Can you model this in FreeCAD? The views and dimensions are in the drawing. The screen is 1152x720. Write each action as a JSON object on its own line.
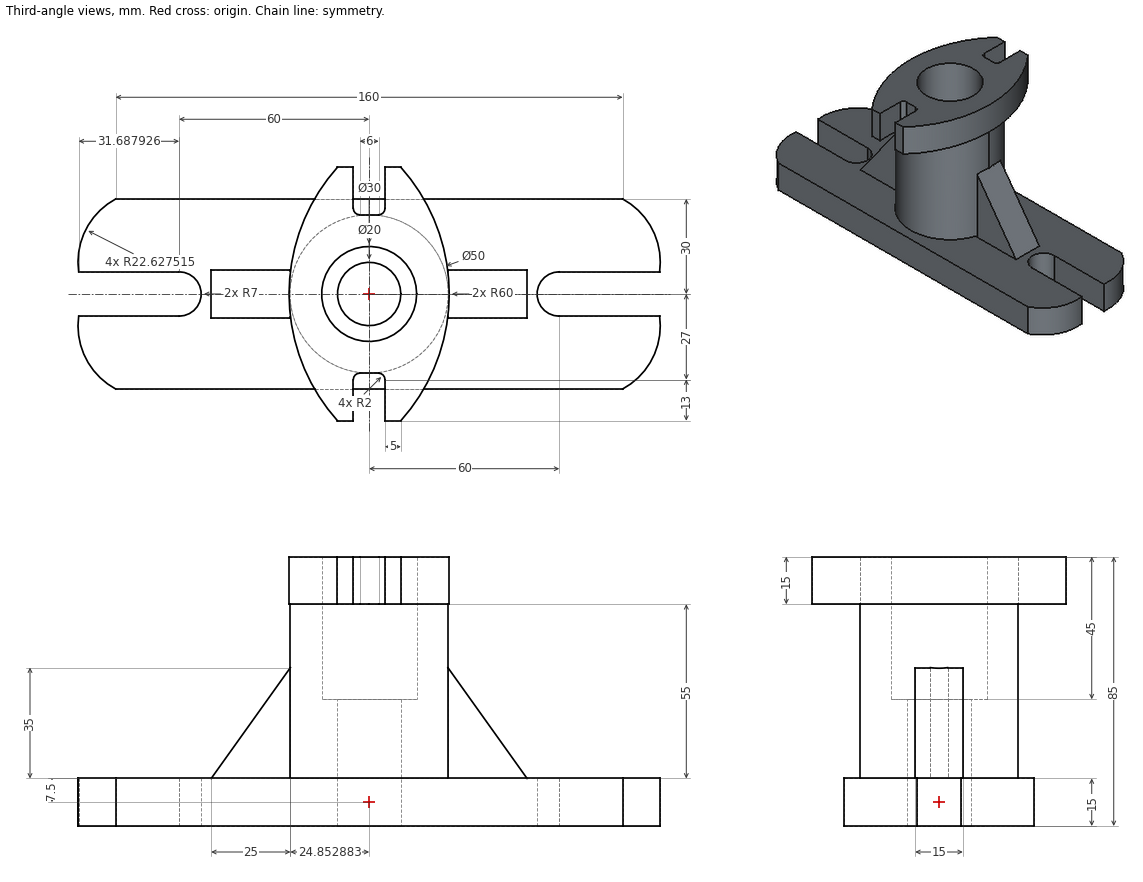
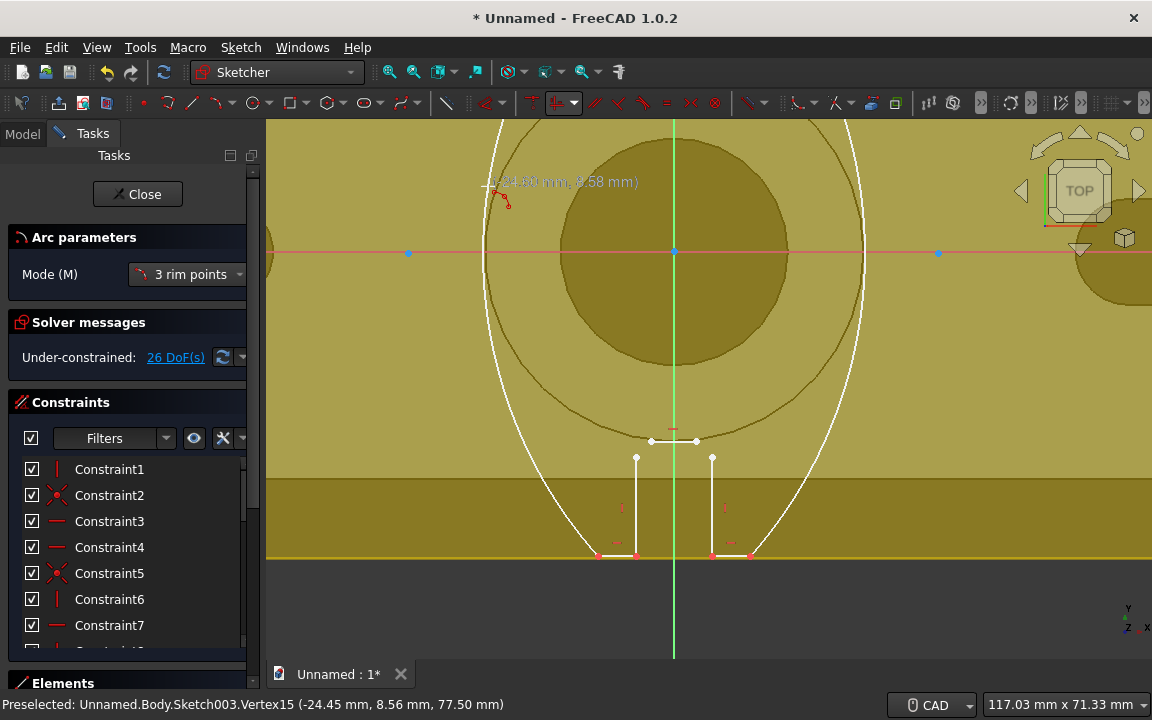
{"action": "left_click", "coordinate": [636, 458]}
{"action": "left_click", "coordinate": [651, 442]}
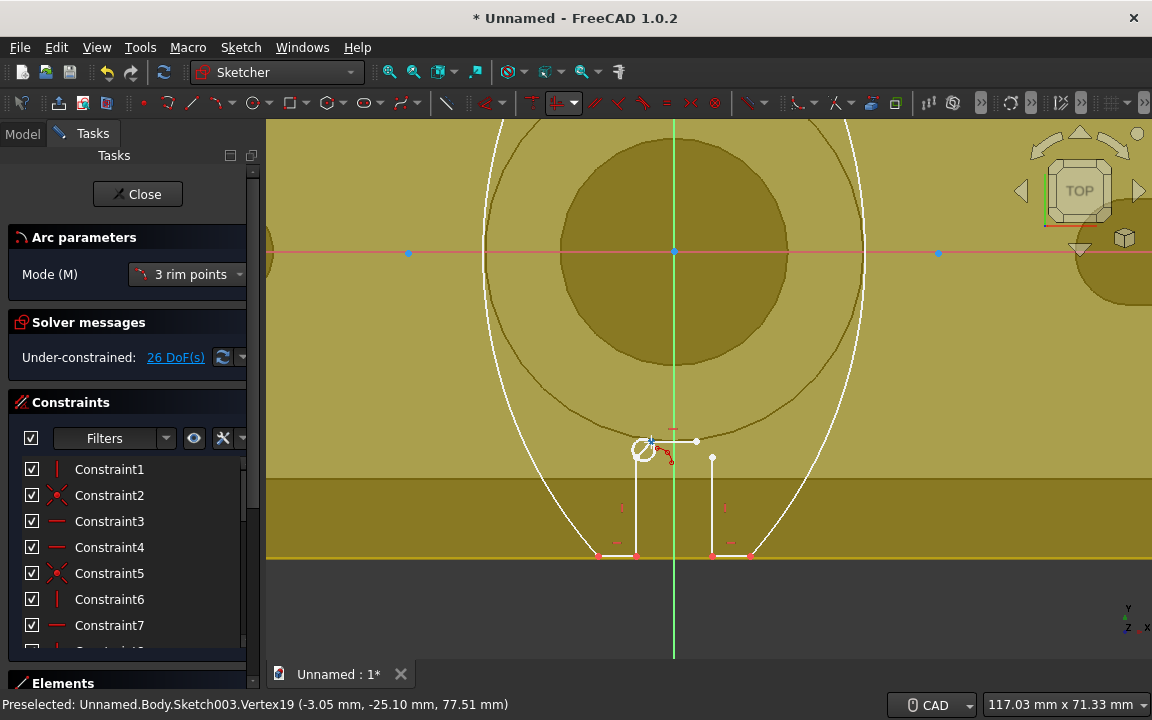
{"action": "scroll", "coordinate": [641, 446], "scroll_direction": "up", "scroll_amount": 7}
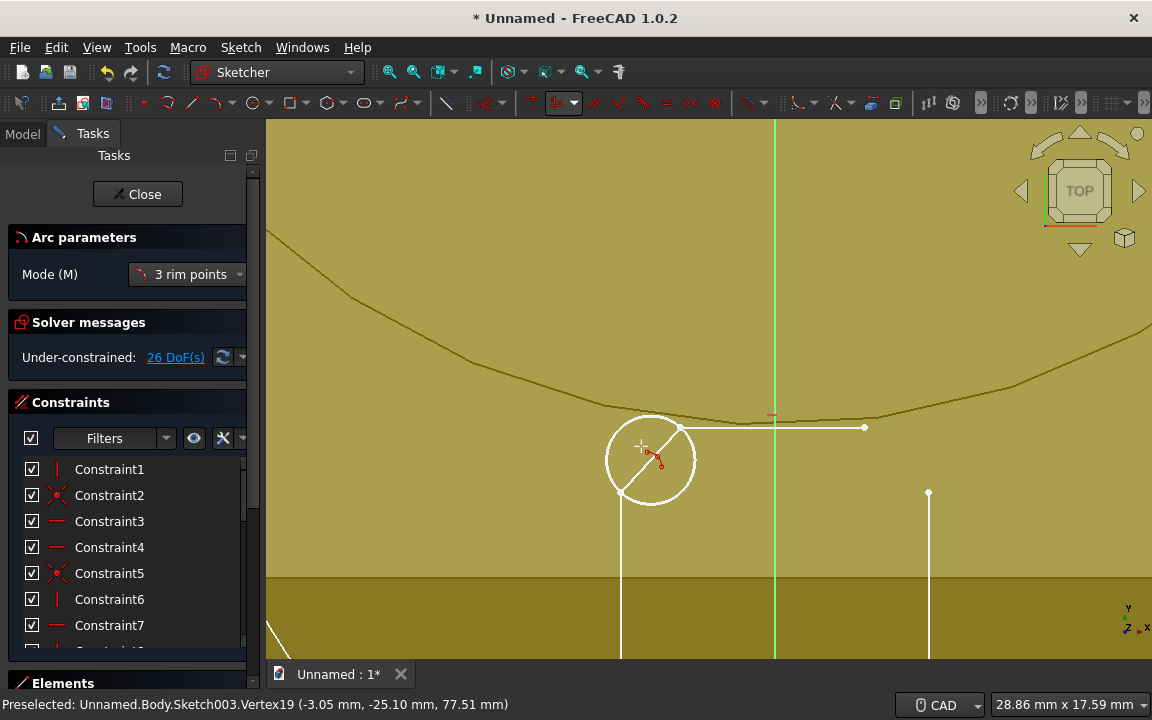
{"action": "left_click", "coordinate": [639, 443]}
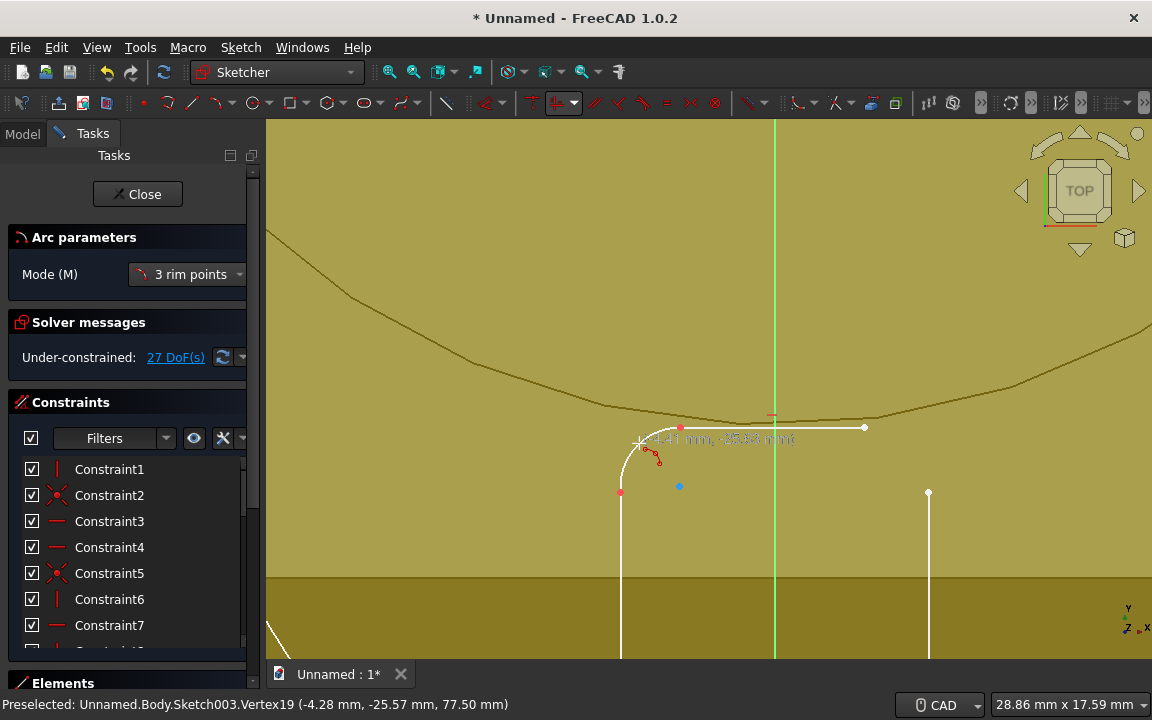
{"action": "scroll", "coordinate": [620, 504], "scroll_direction": "down", "scroll_amount": 10}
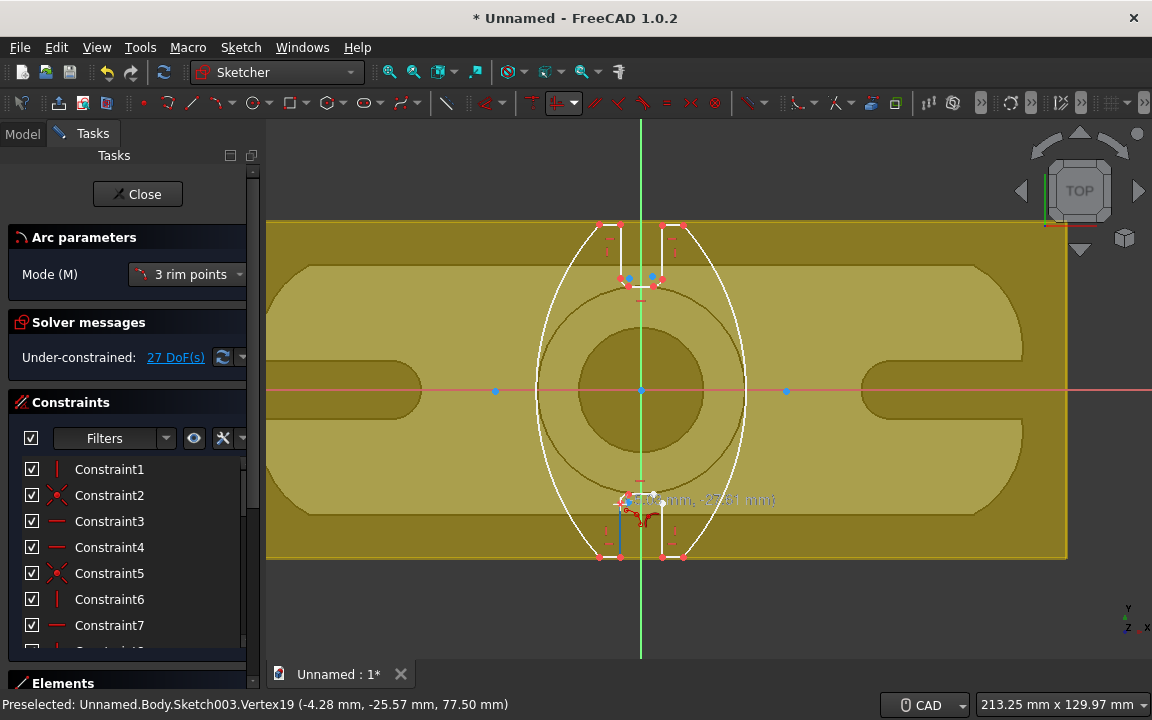
{"action": "scroll", "coordinate": [654, 494], "scroll_direction": "up", "scroll_amount": 2}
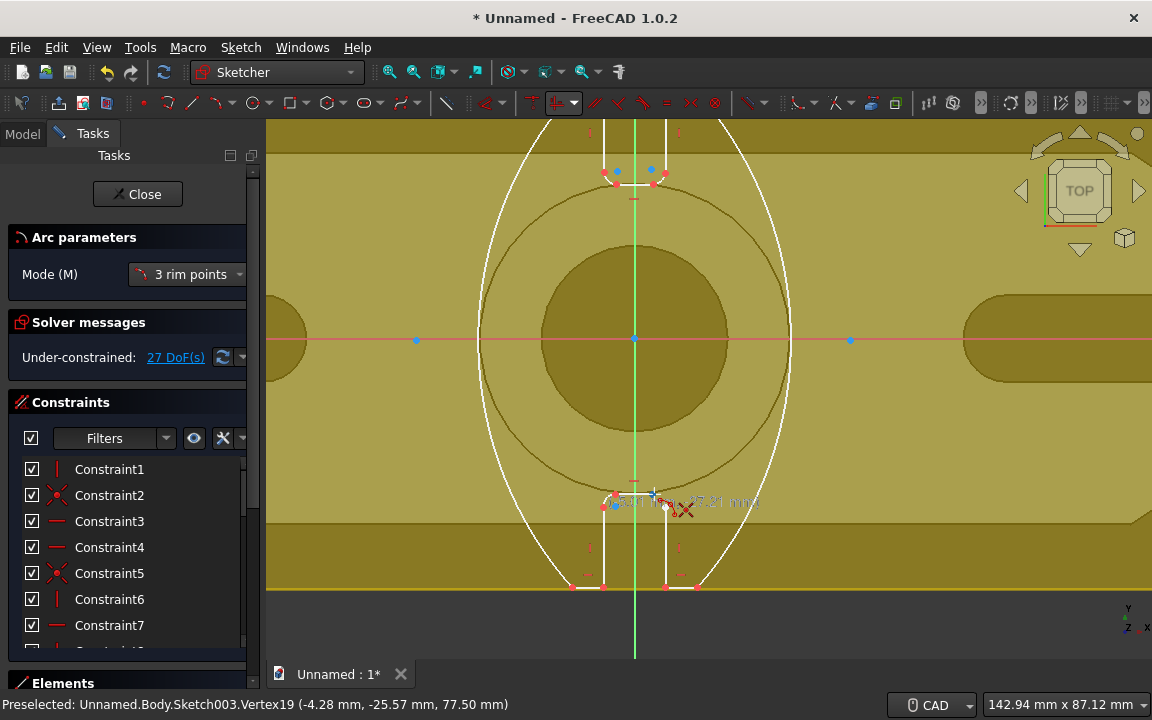
{"action": "left_click", "coordinate": [653, 494]}
{"action": "left_click", "coordinate": [666, 507]}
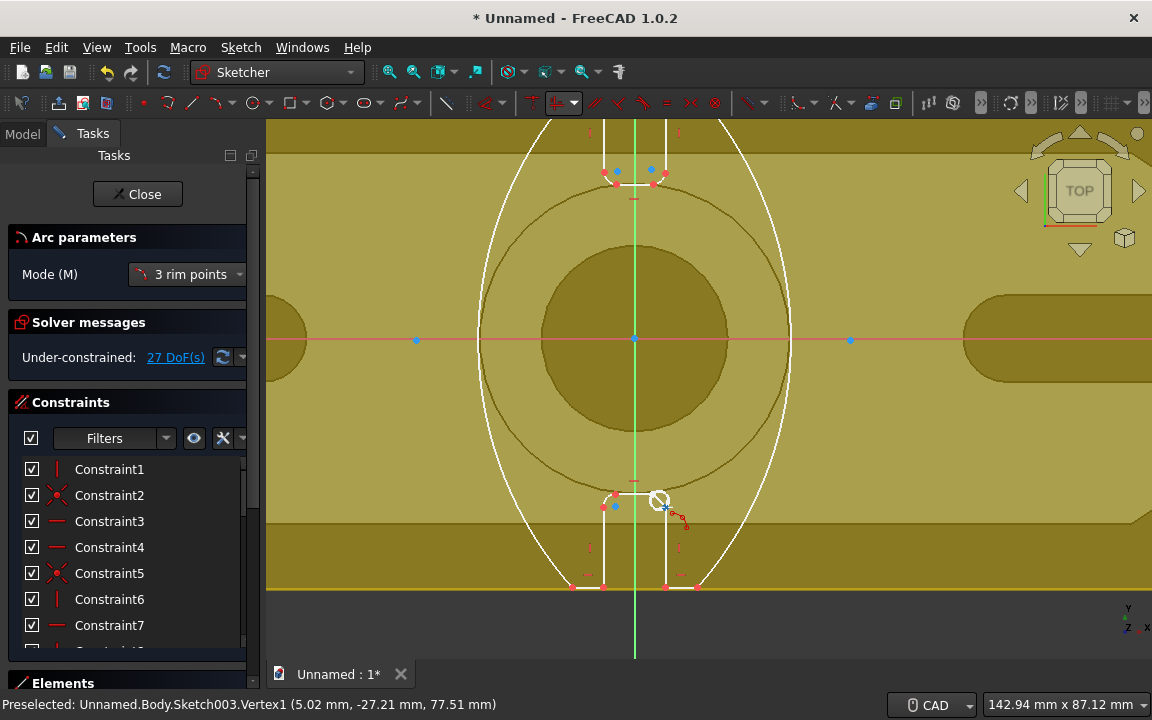
{"action": "scroll", "coordinate": [662, 497], "scroll_direction": "up", "scroll_amount": 8}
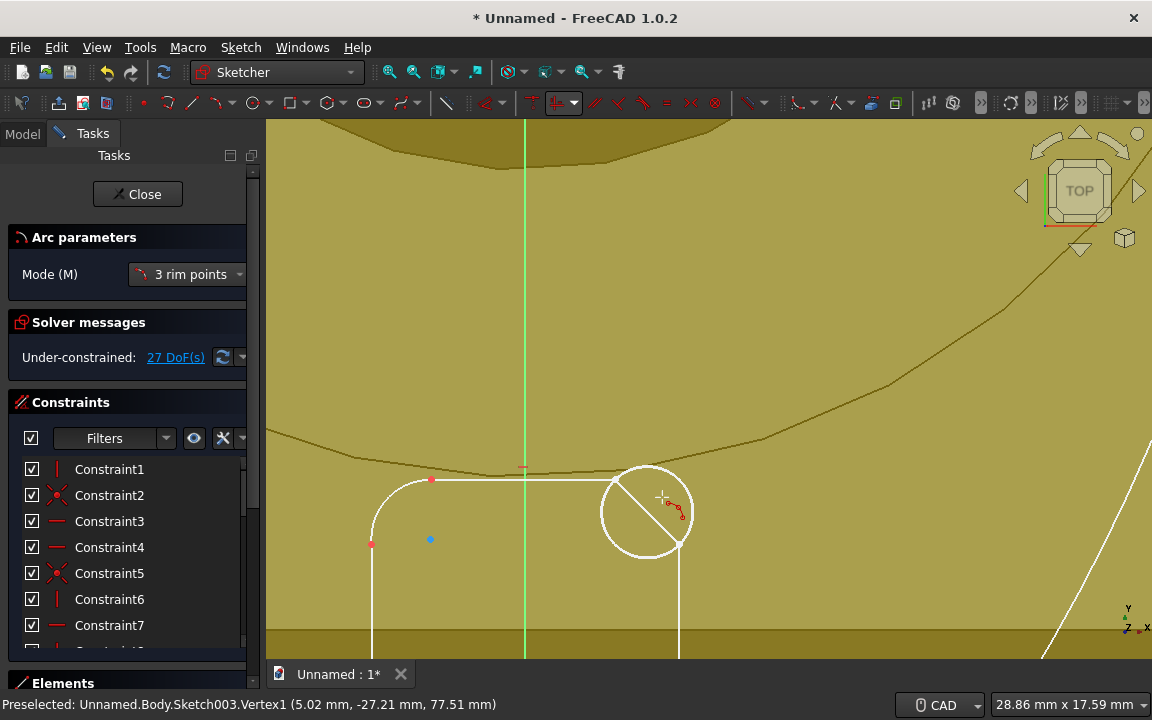
{"action": "left_click", "coordinate": [661, 495]}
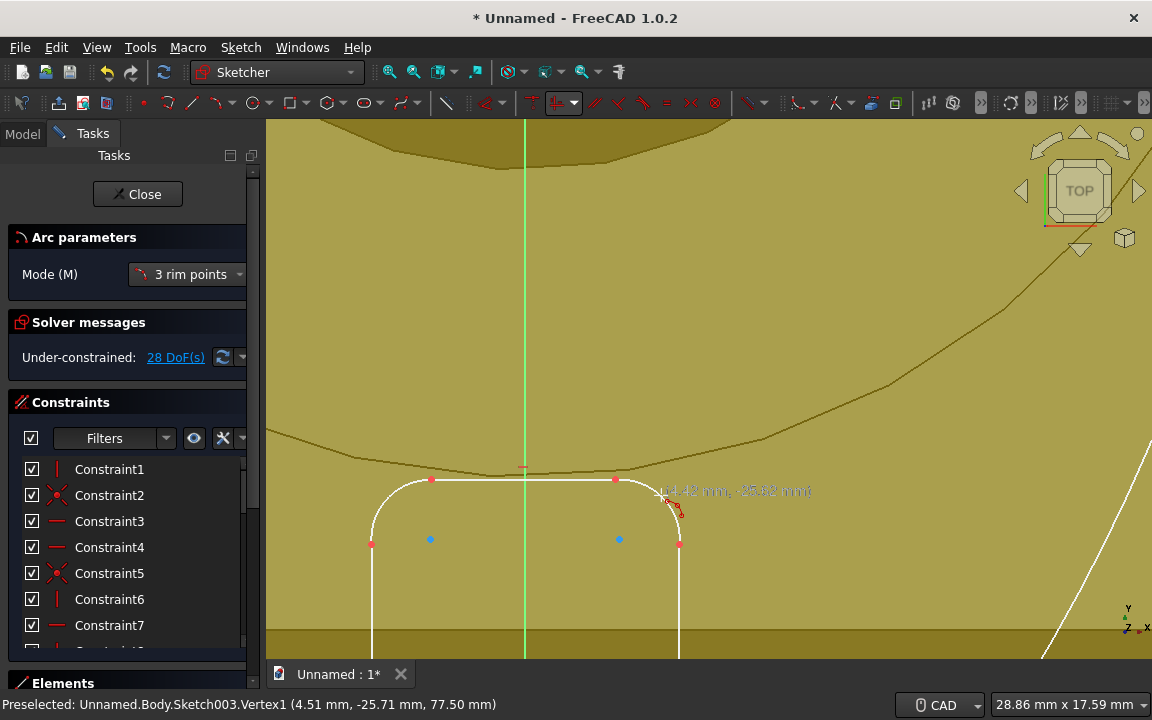
{"action": "left_click", "coordinate": [254, 104]}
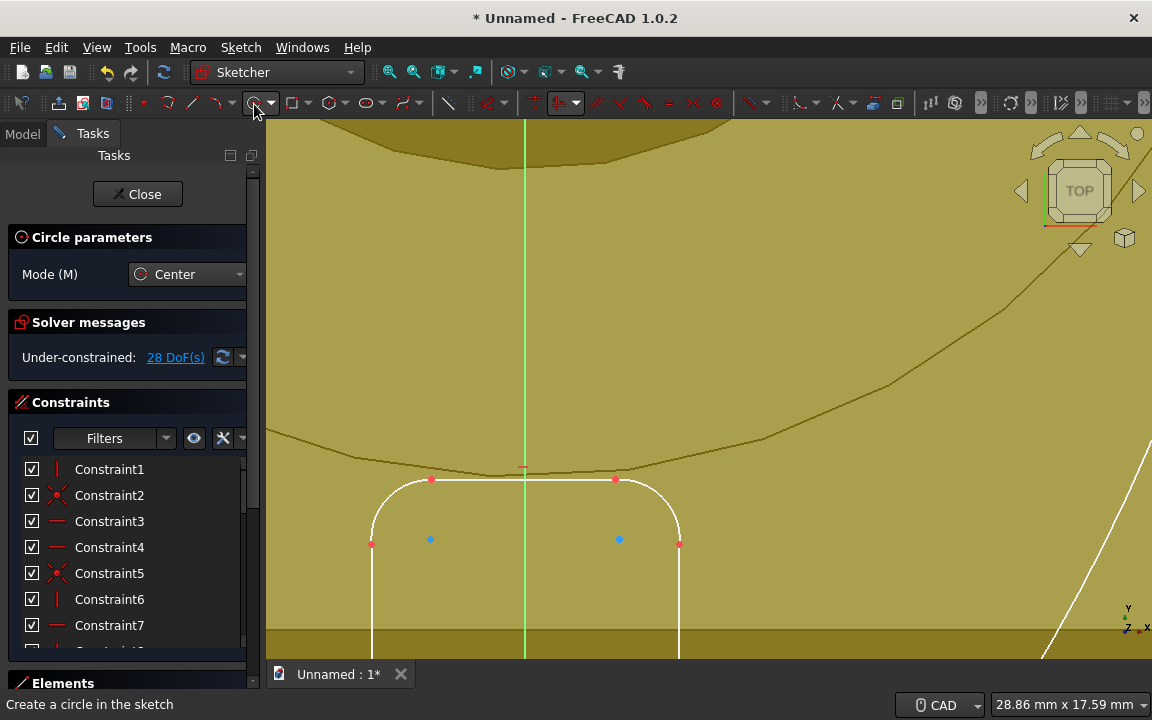
{"action": "scroll", "coordinate": [659, 495], "scroll_direction": "down", "scroll_amount": 10}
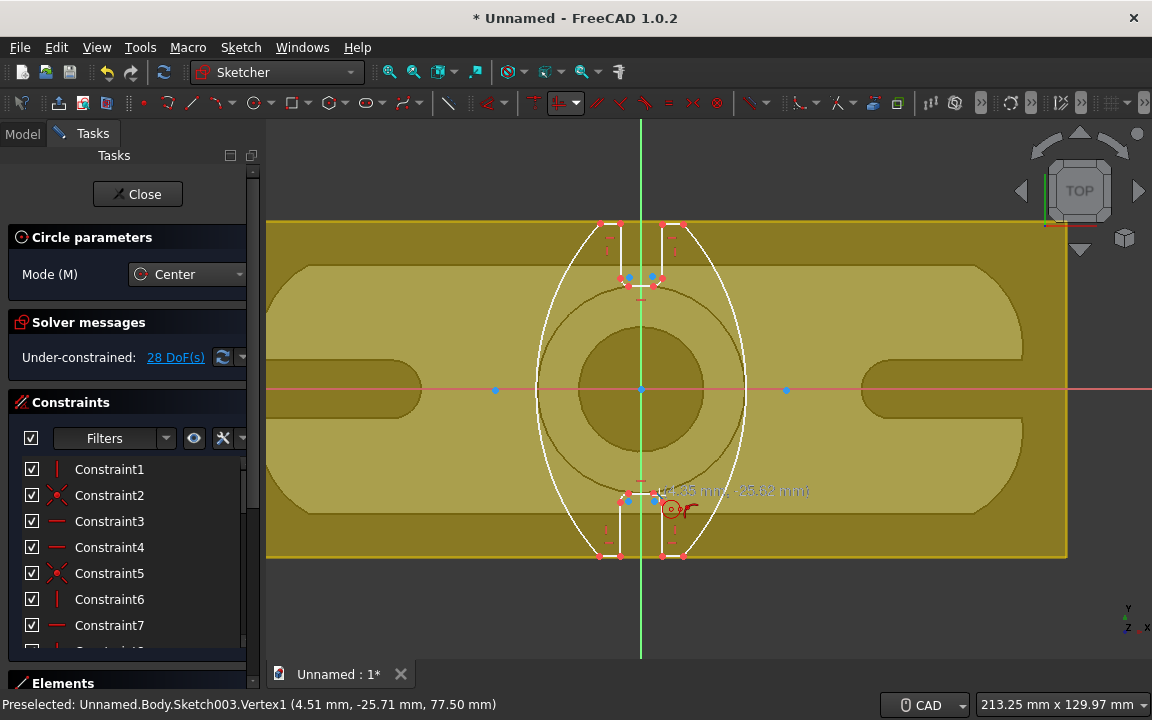
{"action": "left_click", "coordinate": [641, 389]}
{"action": "mouse_move", "coordinate": [685, 345]}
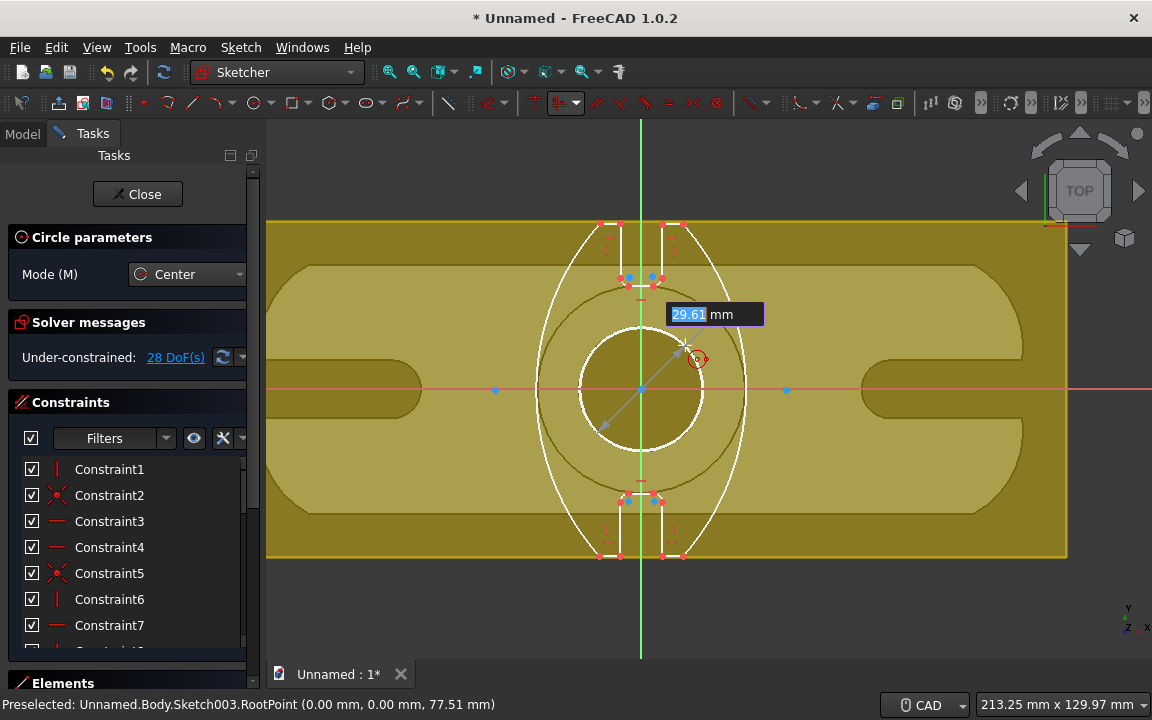
{"action": "type", "text": "30"}
{"action": "key", "text": "Return"}
{"action": "key", "text": "Escape"}